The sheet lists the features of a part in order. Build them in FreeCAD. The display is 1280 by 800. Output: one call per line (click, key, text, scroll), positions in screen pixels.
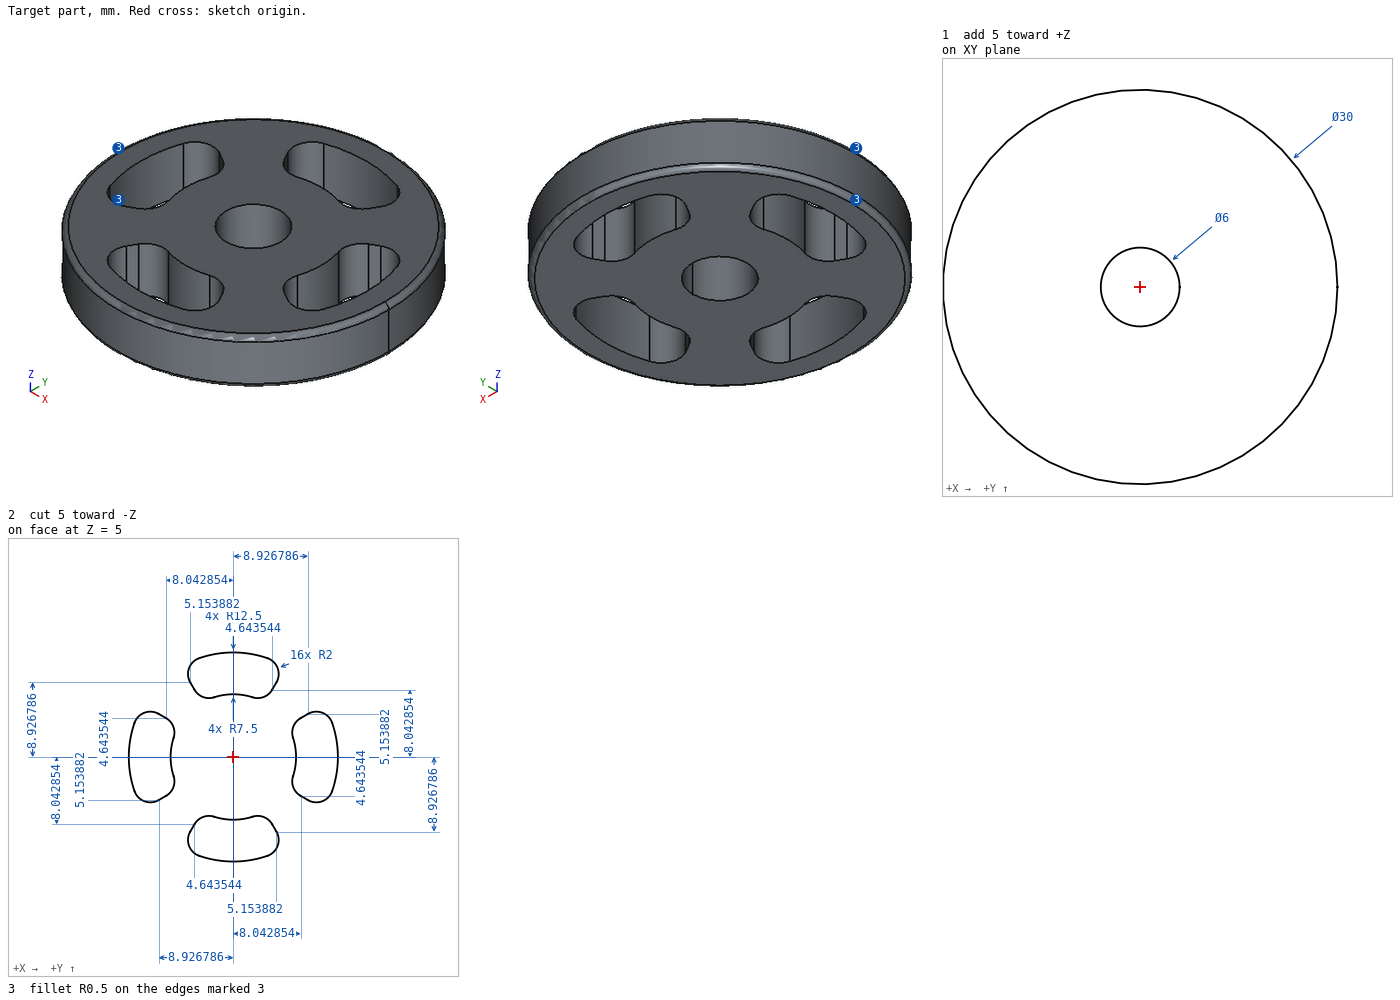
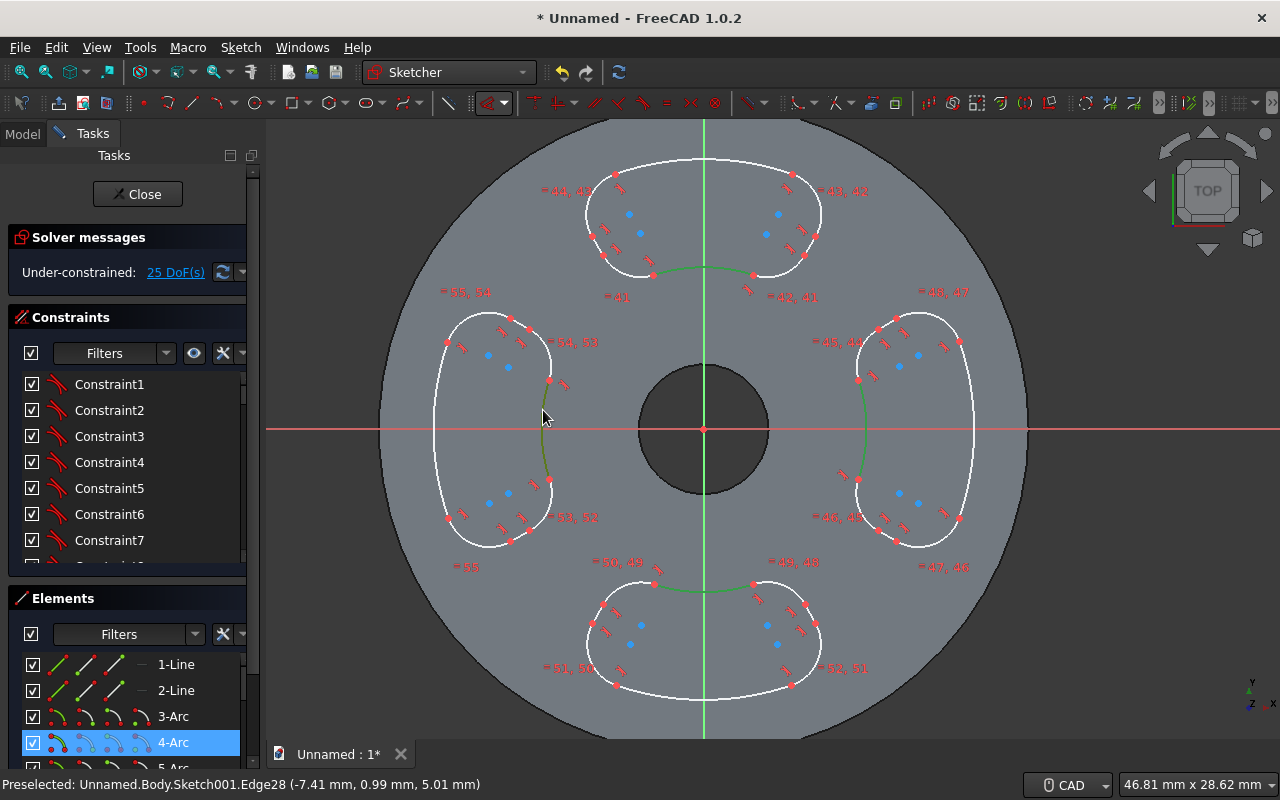
click(668, 104)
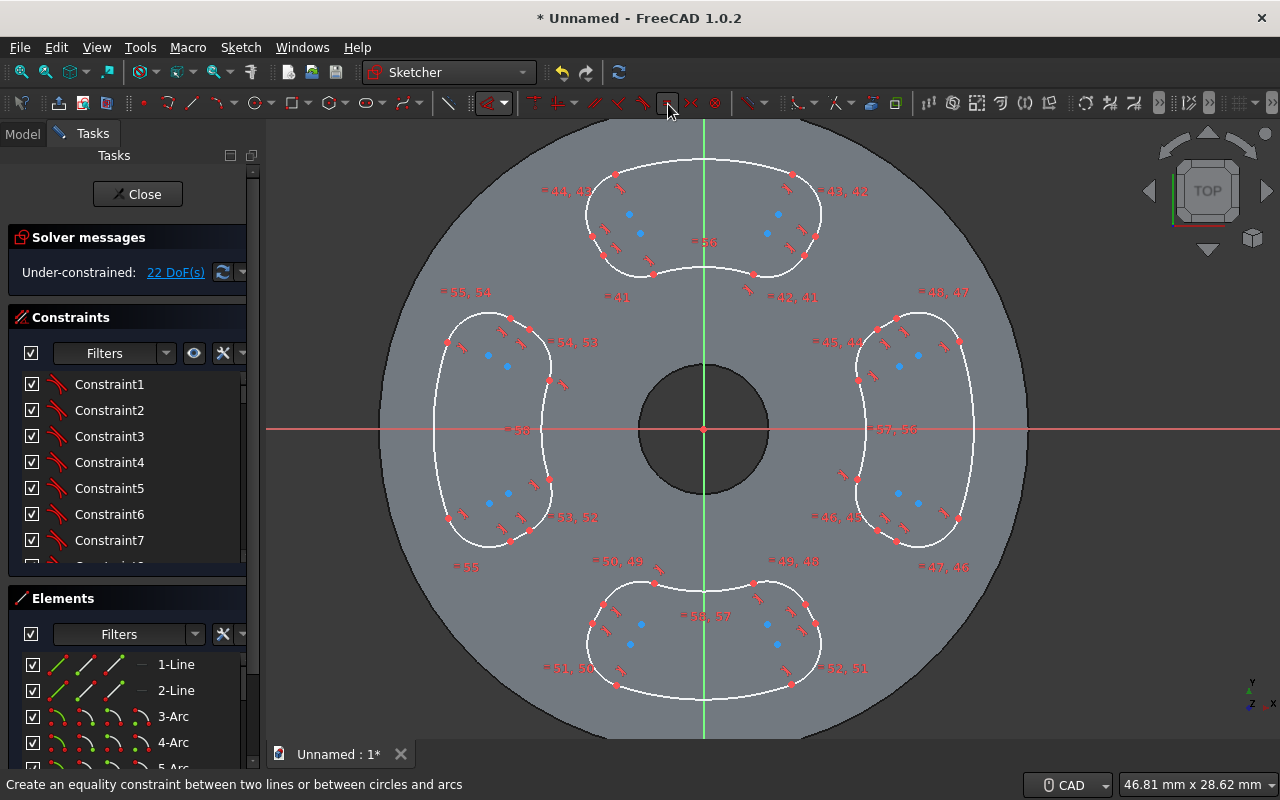
click(740, 162)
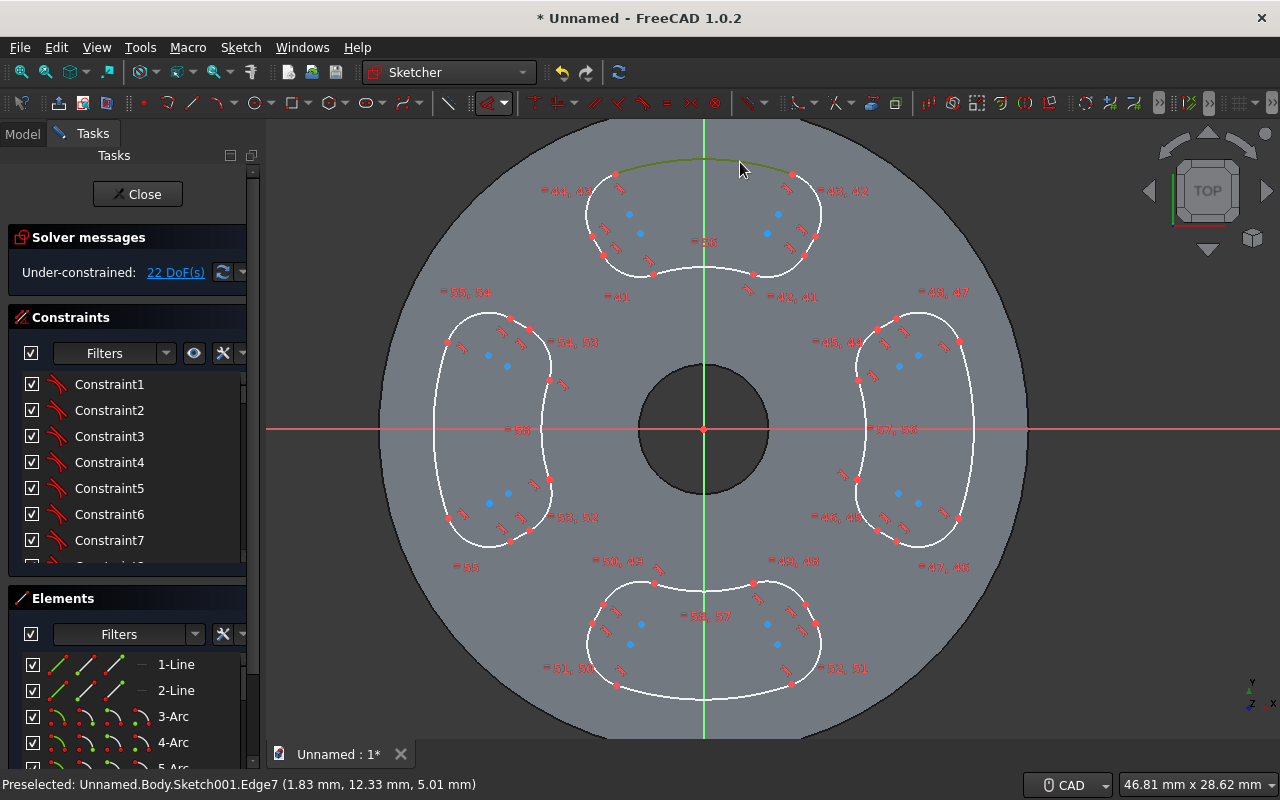
click(971, 466)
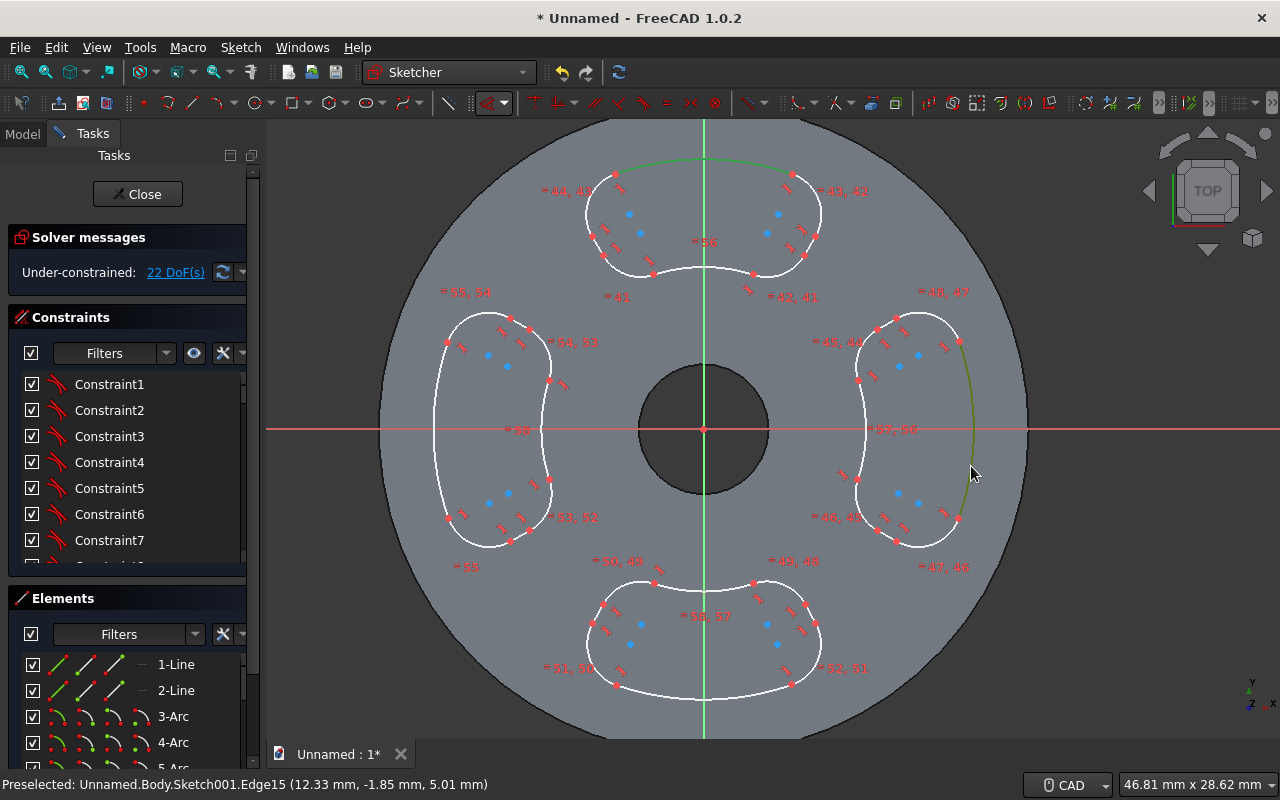
click(669, 697)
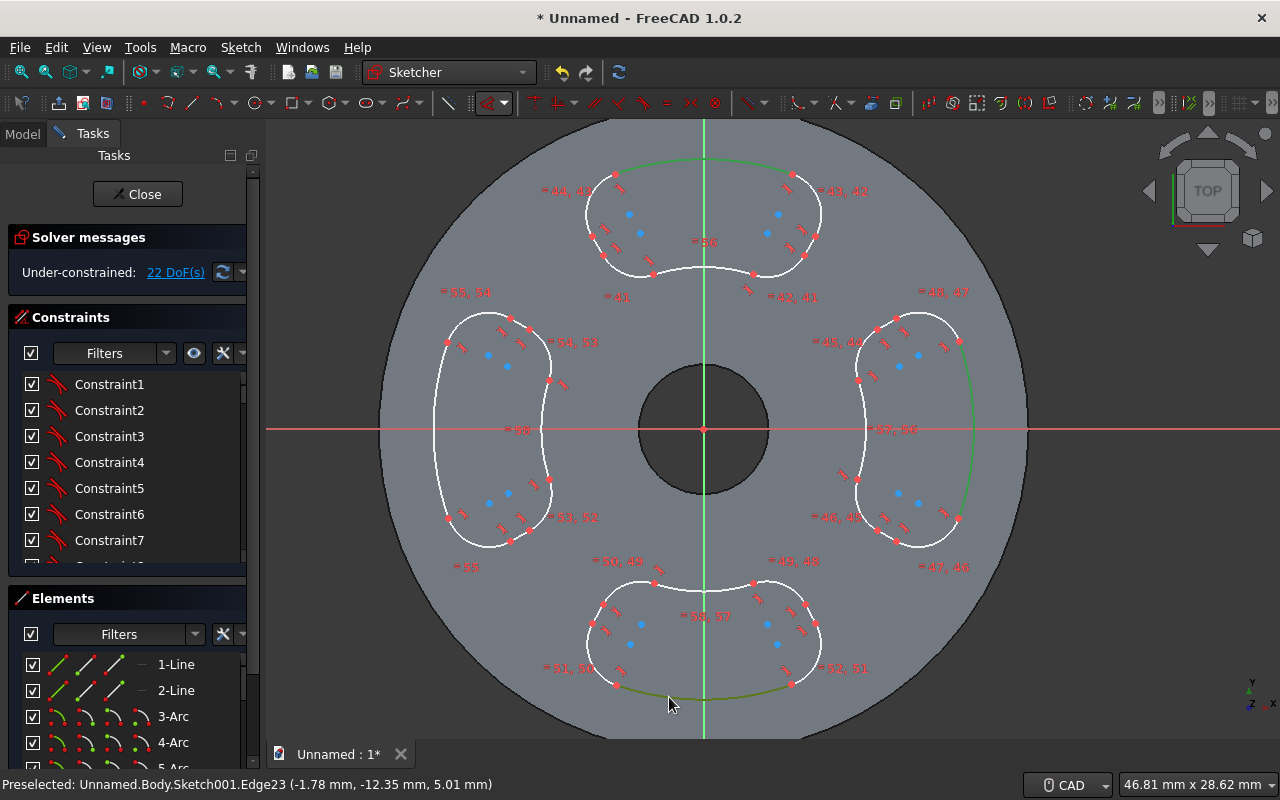
click(436, 394)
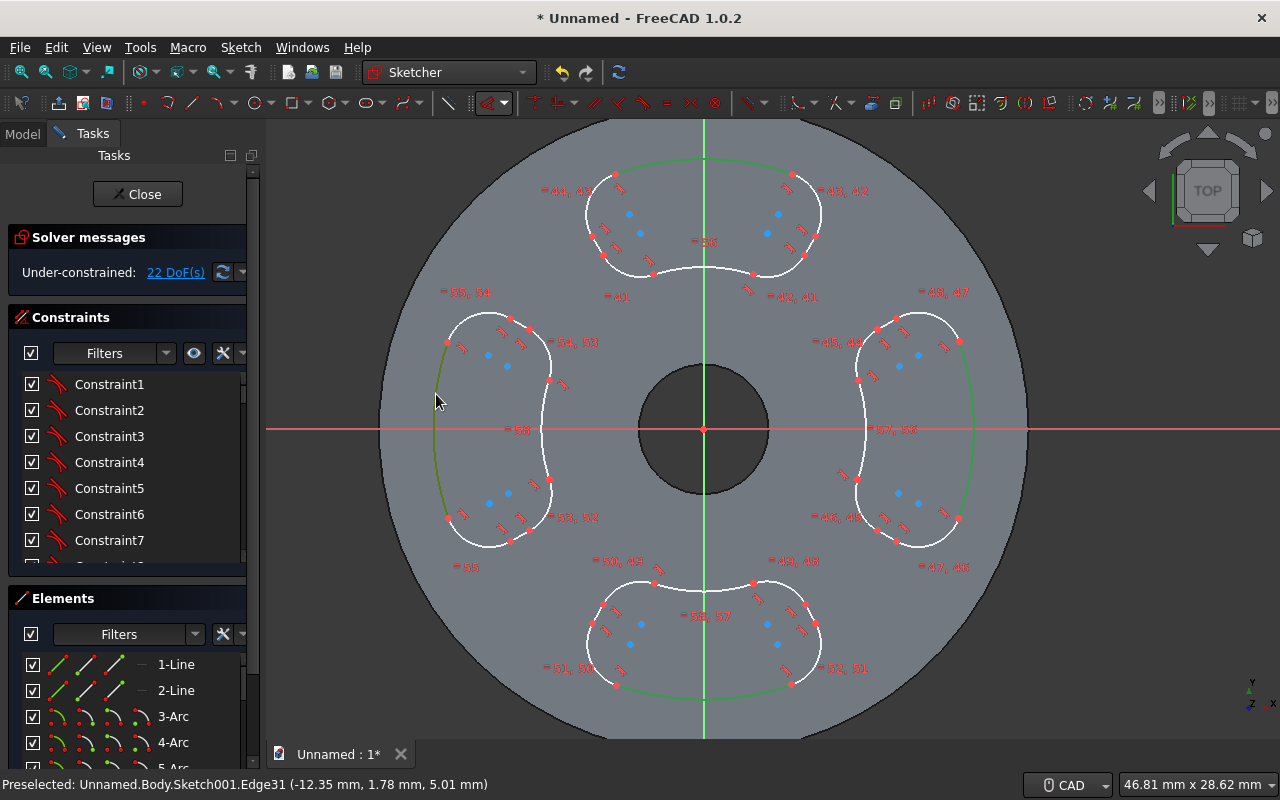
click(668, 104)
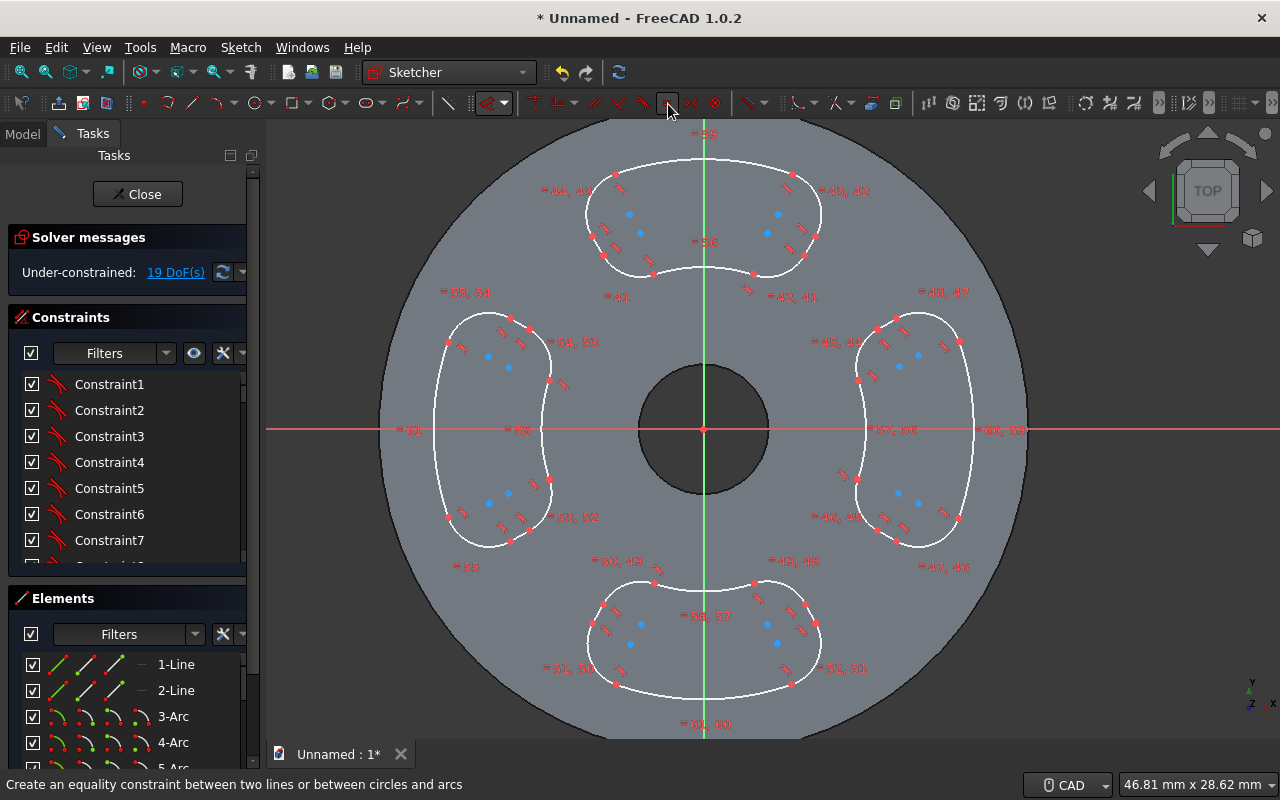
click(615, 269)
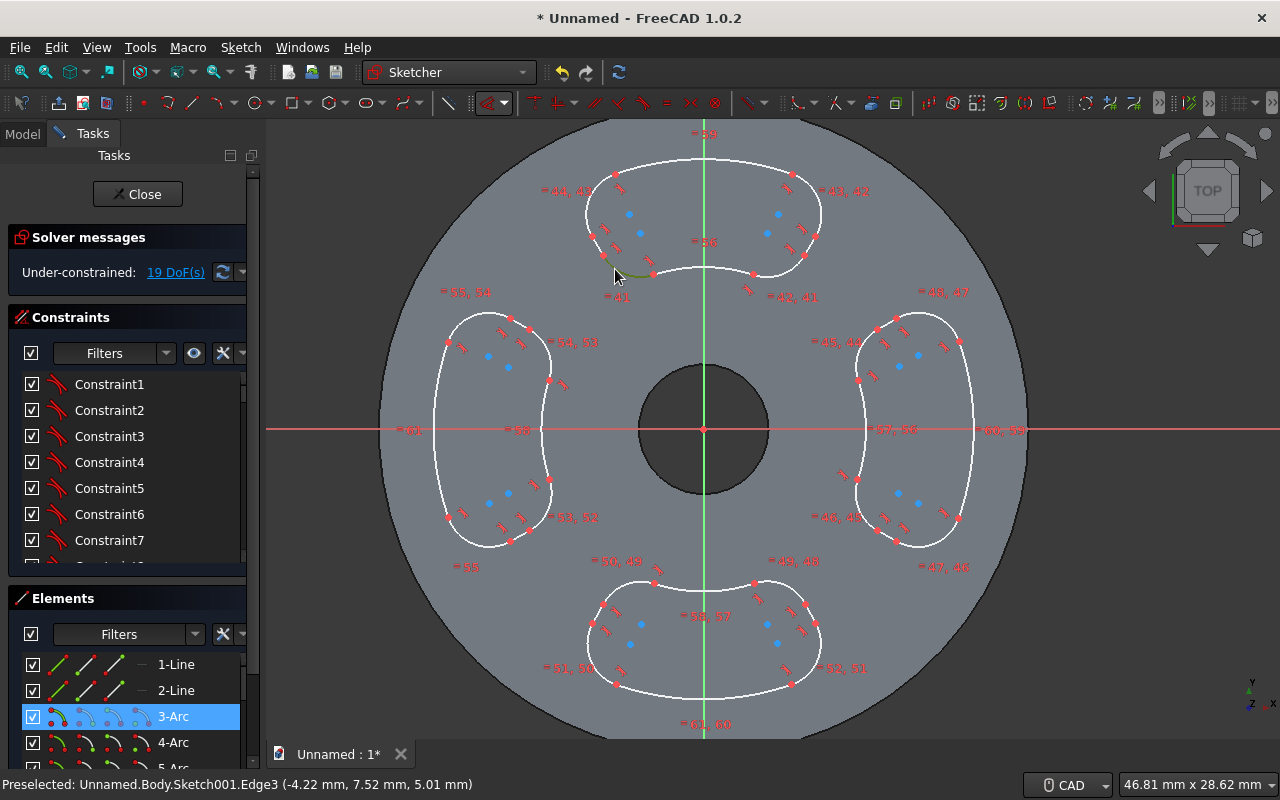
key(k)
key(r)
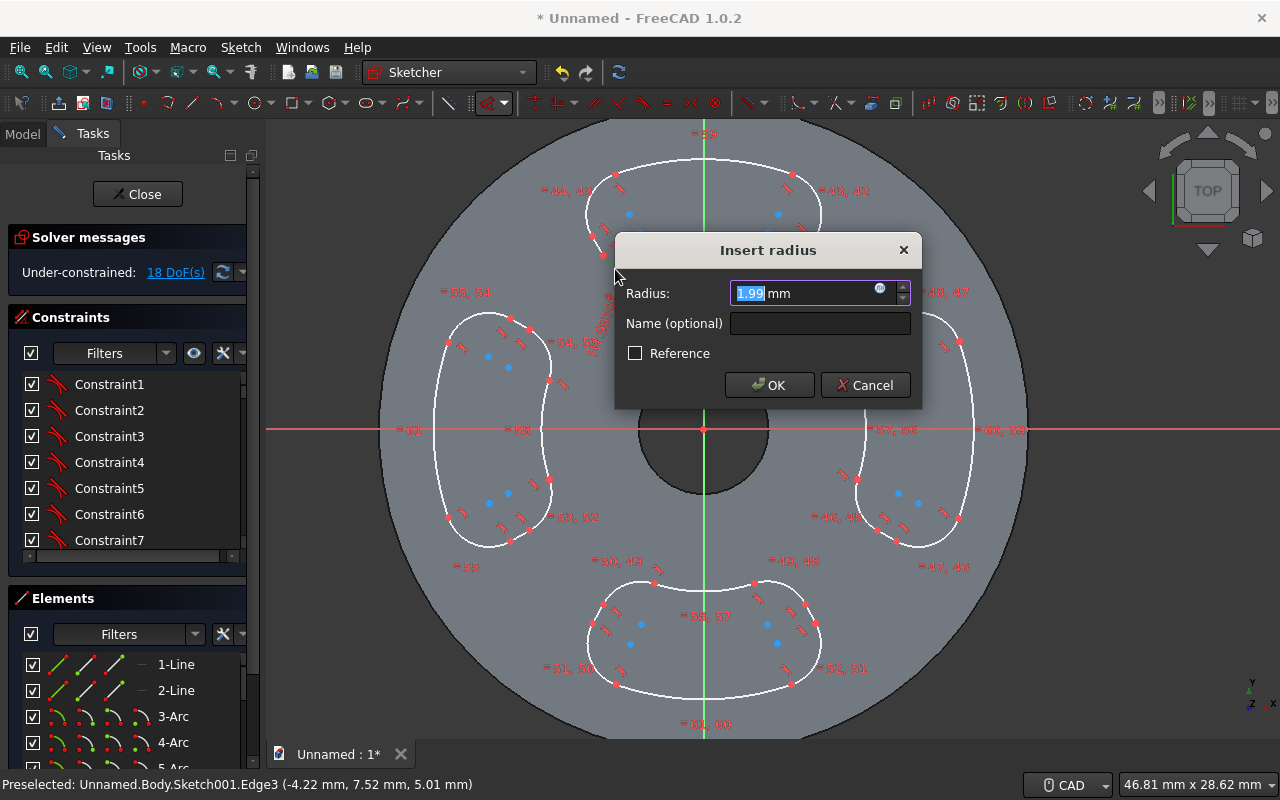
text(2)
key(Return)